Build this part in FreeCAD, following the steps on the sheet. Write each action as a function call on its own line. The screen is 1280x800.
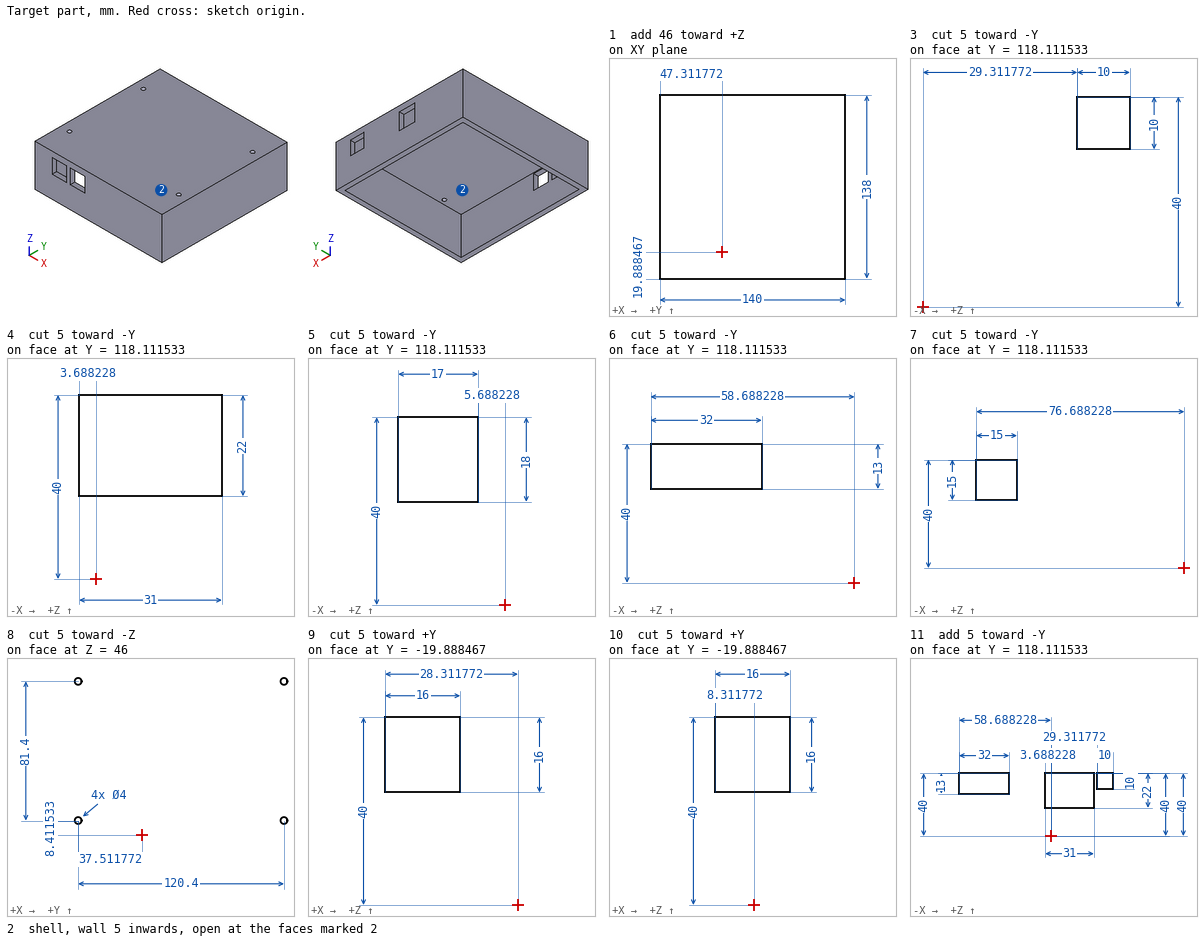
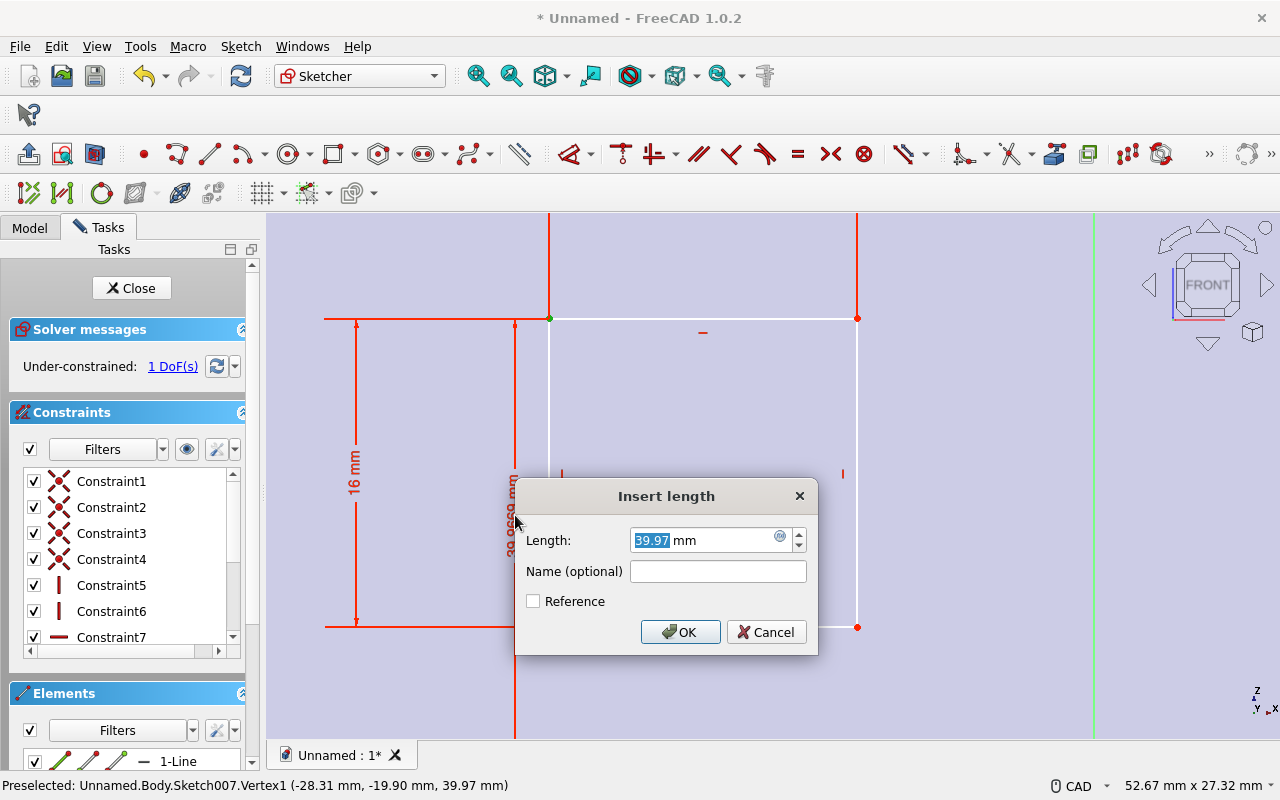
text(40)
key(Return)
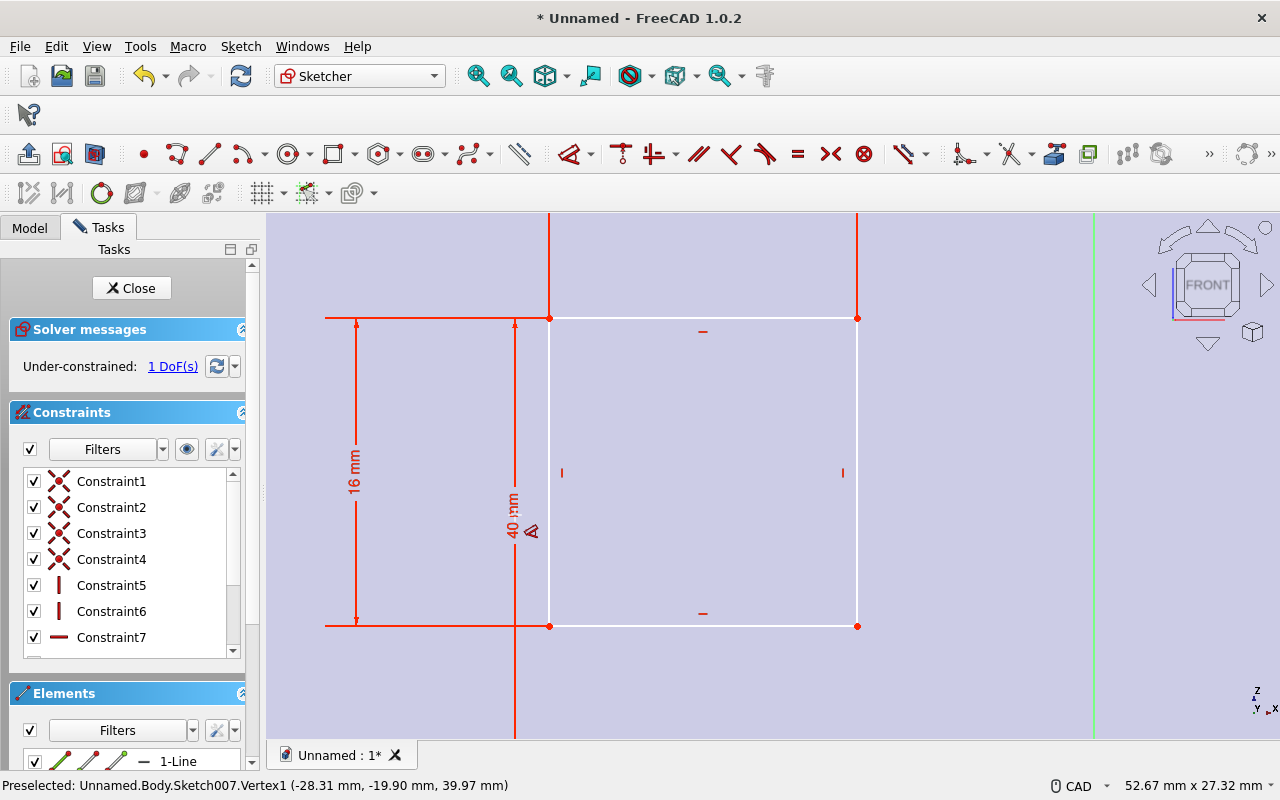
click(549, 318)
click(822, 284)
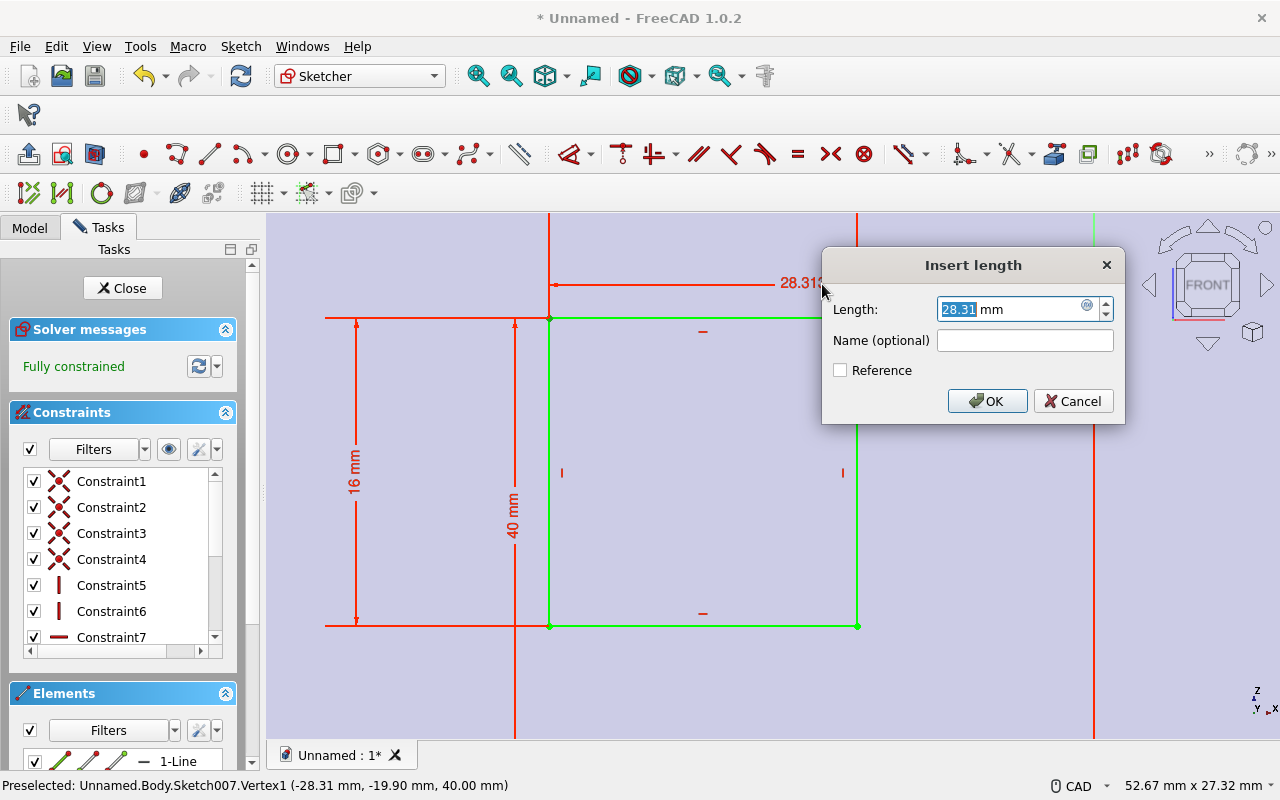
text(28.311772)
key(Return)
key(Escape)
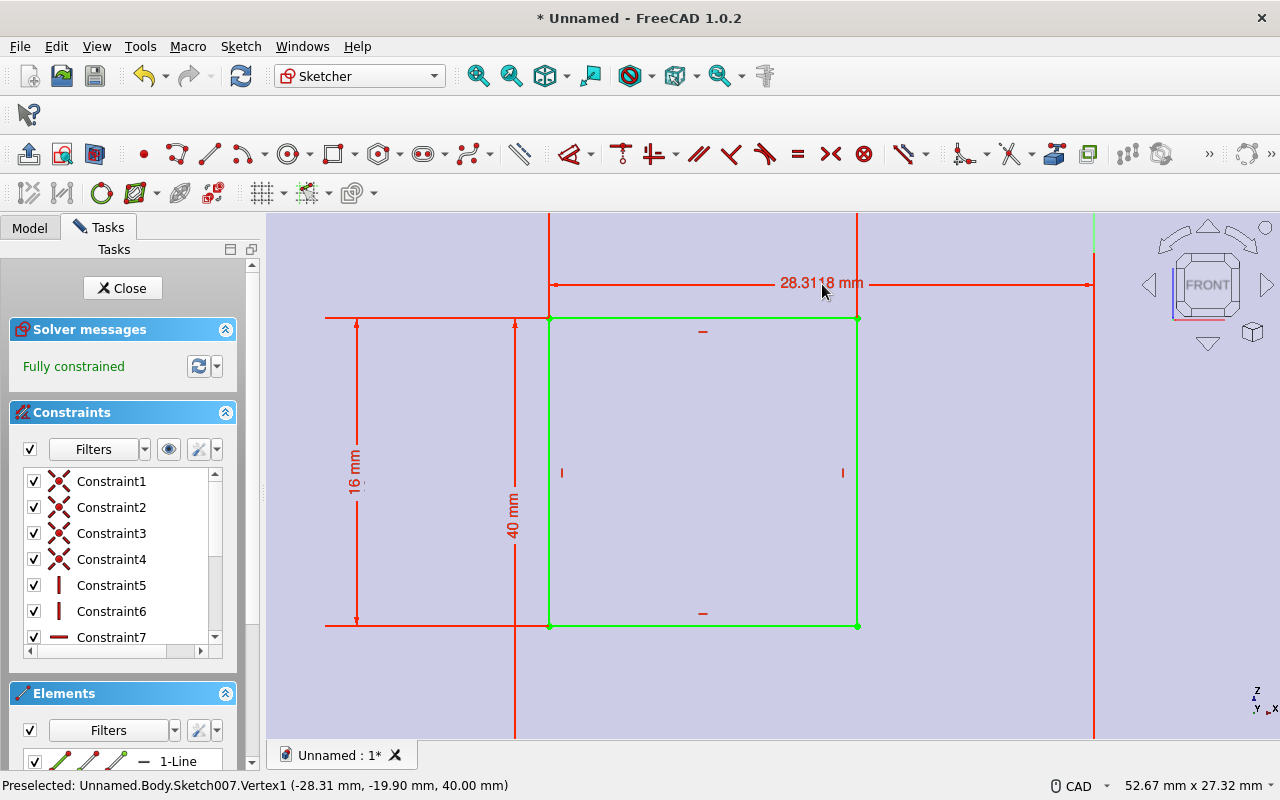
click(123, 288)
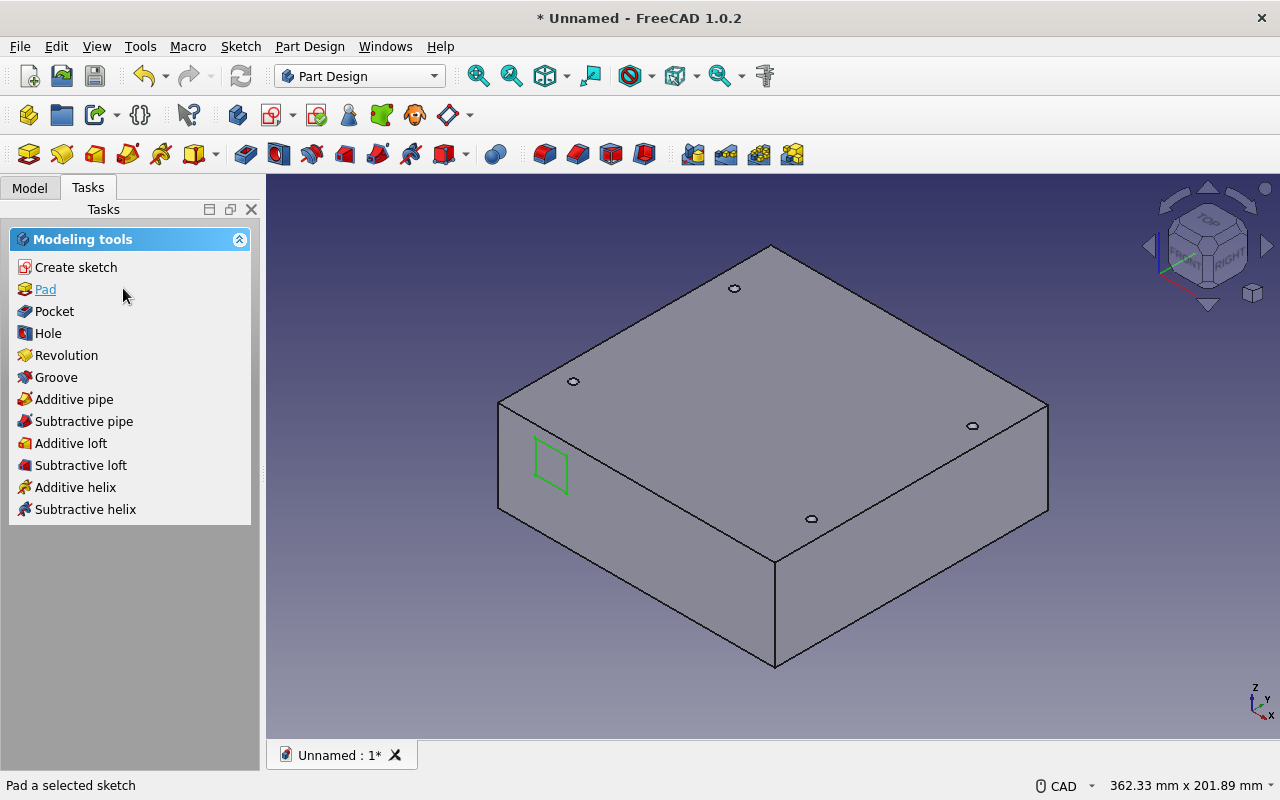
click(246, 154)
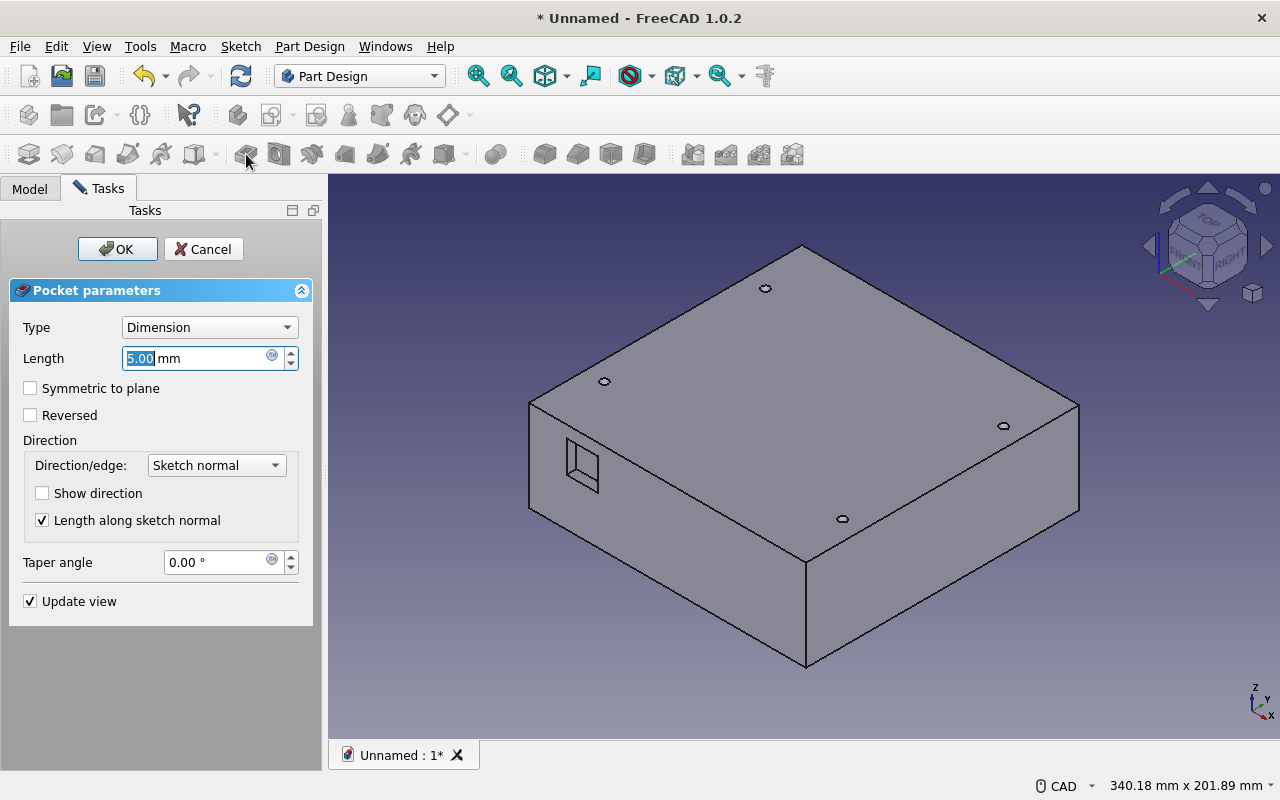
text(5)
key(Tab)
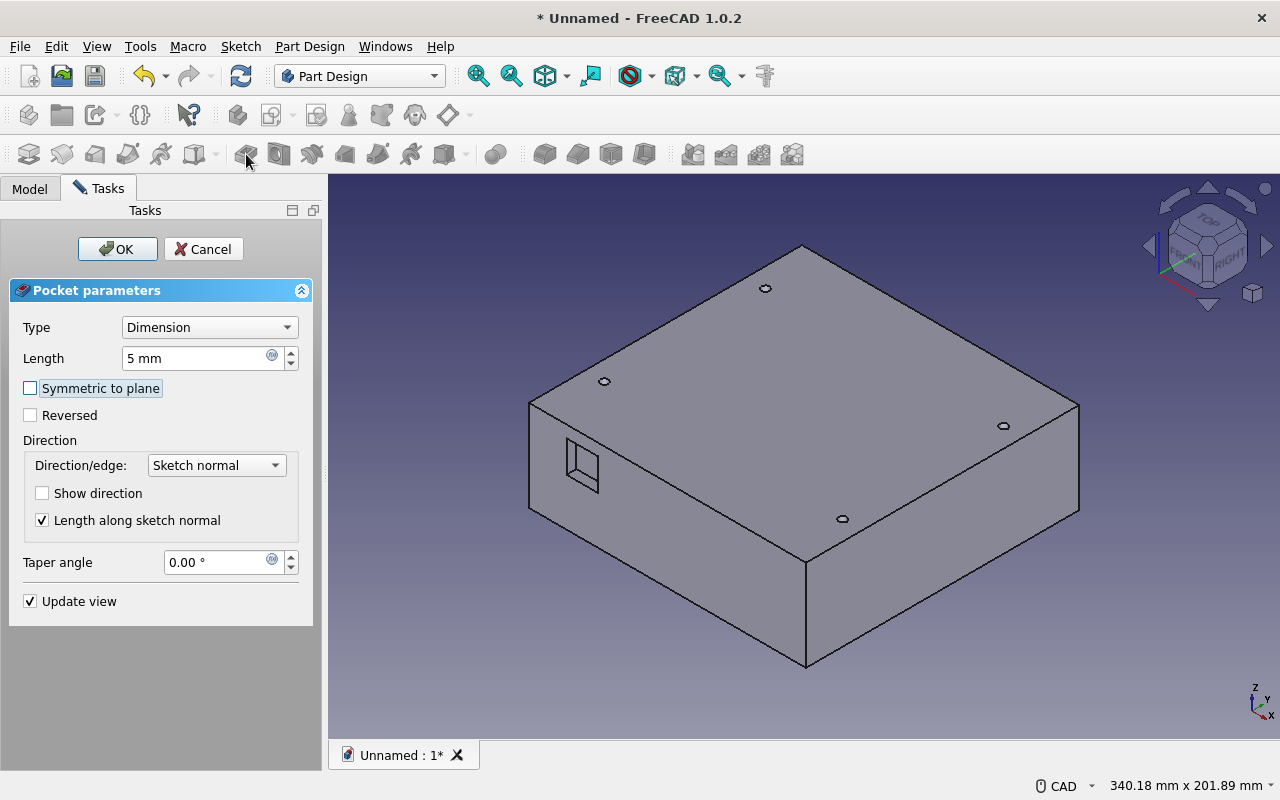
click(118, 249)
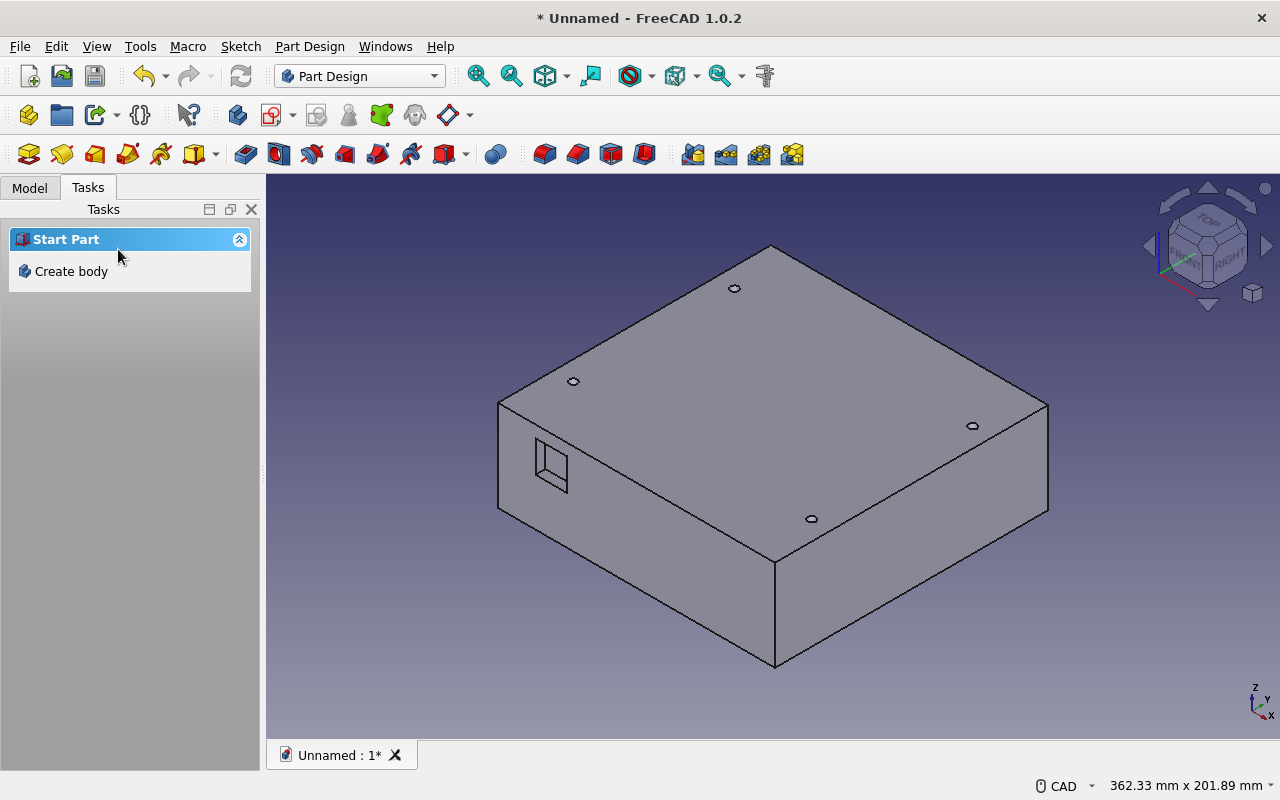
click(716, 580)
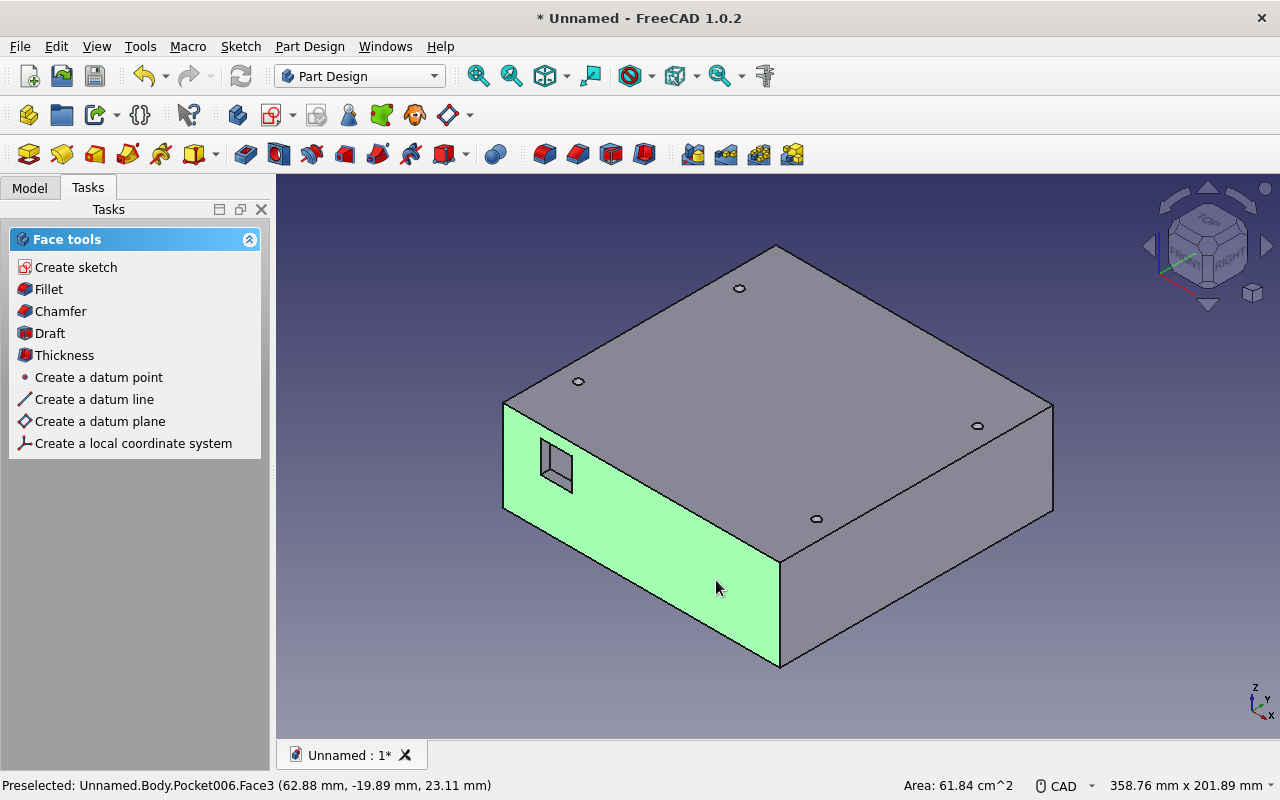
click(270, 116)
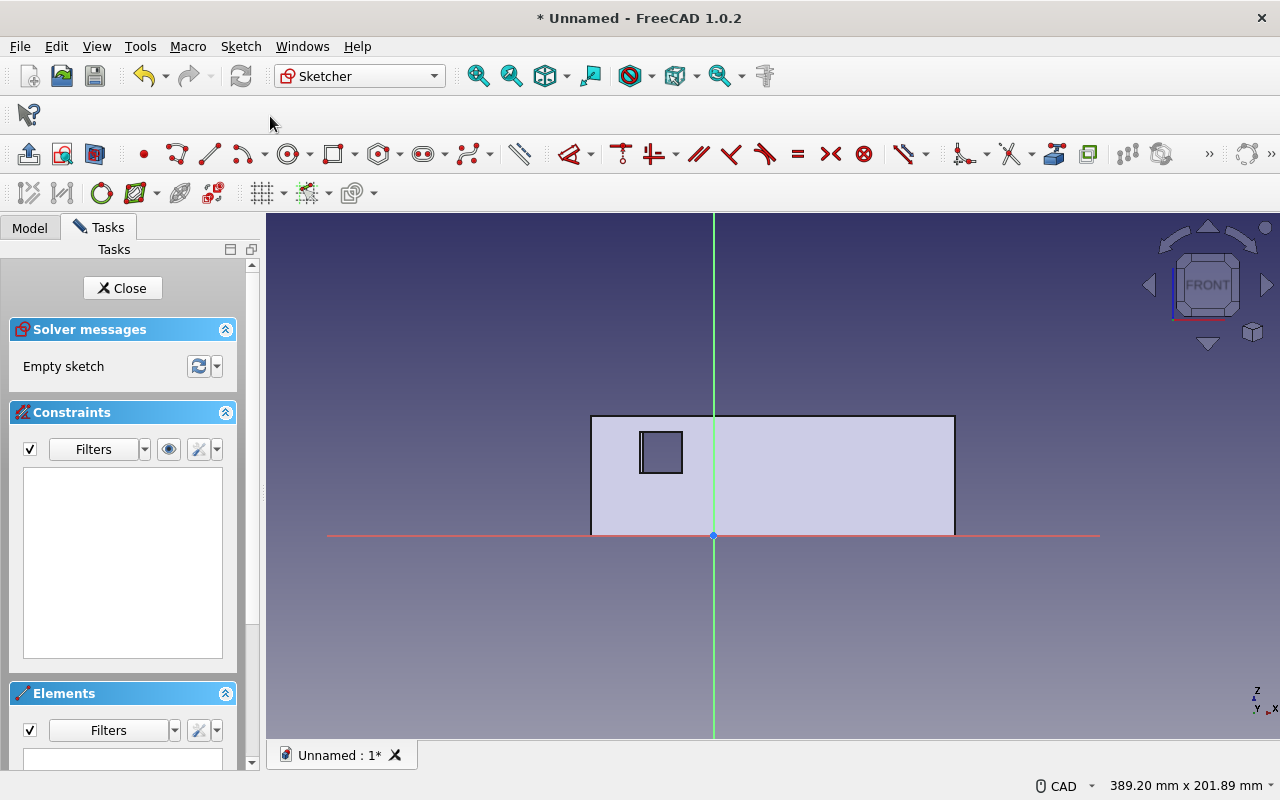
scroll(714, 449, up, 10)